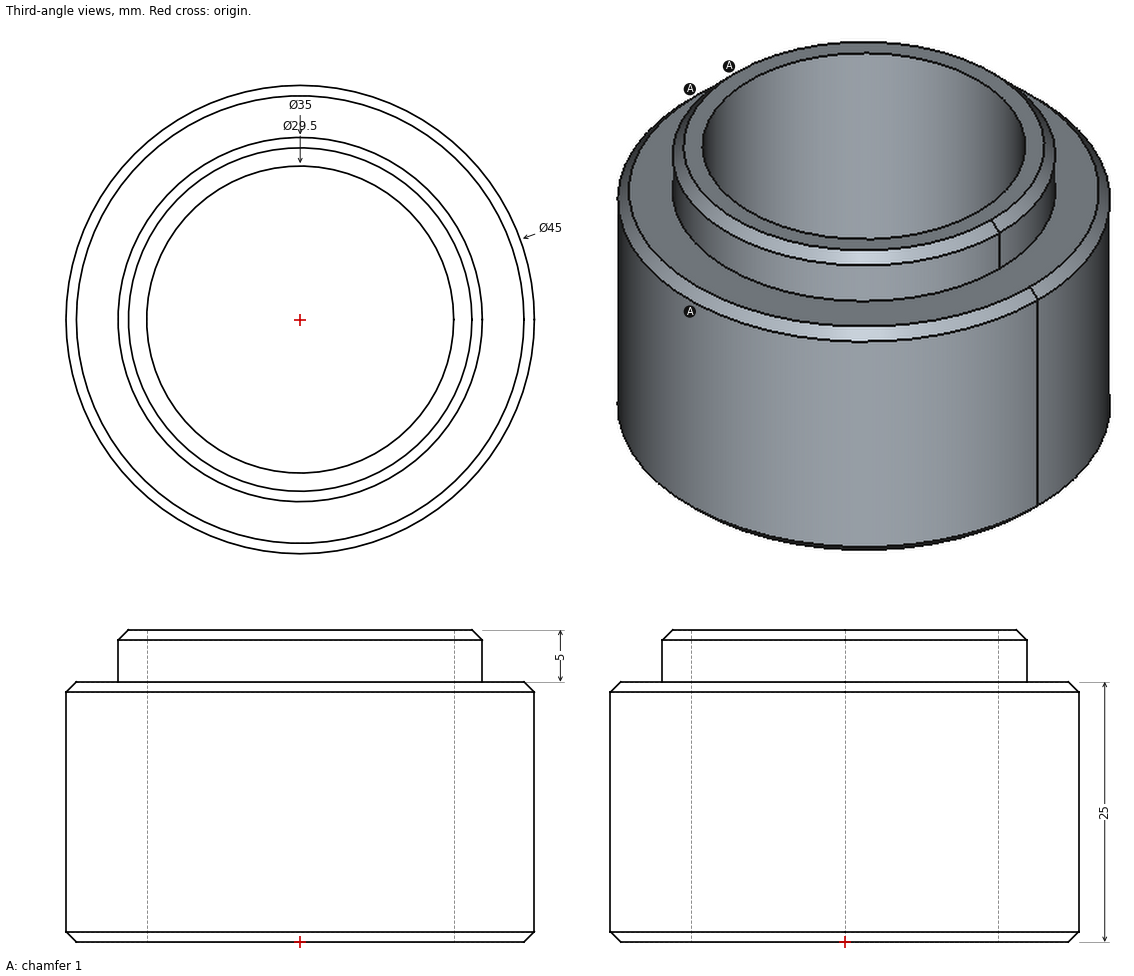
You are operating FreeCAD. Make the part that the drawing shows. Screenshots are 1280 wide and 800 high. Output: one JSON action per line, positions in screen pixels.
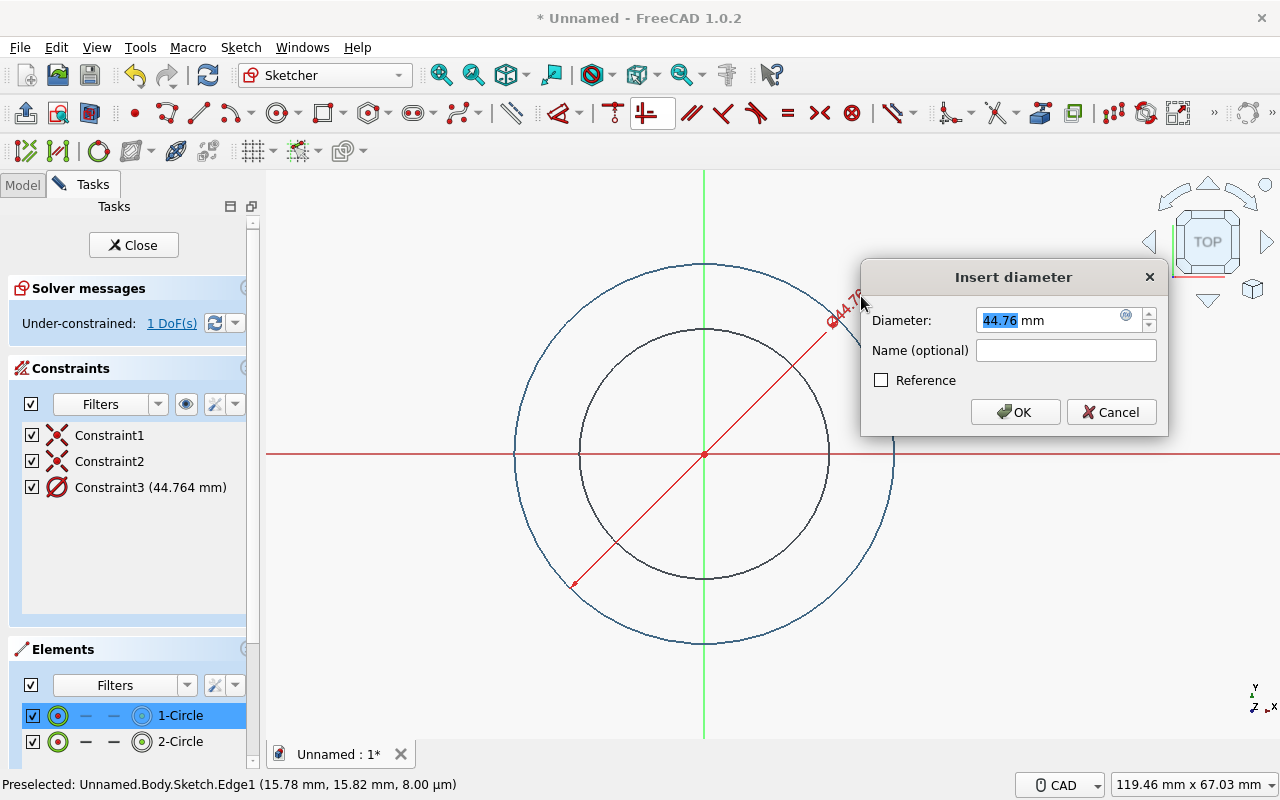
{"action": "type", "text": "45"}
{"action": "key", "text": "Return"}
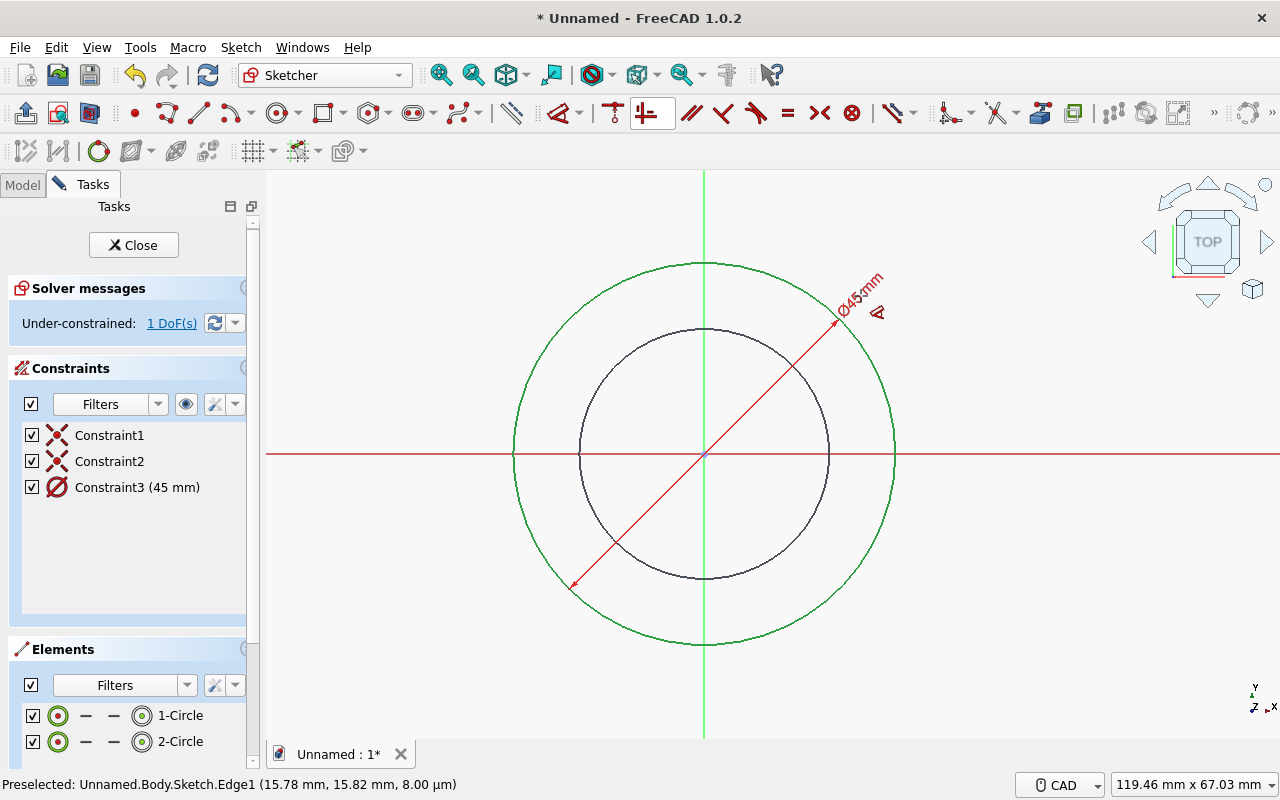
{"action": "left_click", "coordinate": [792, 365]}
{"action": "left_click", "coordinate": [814, 342]}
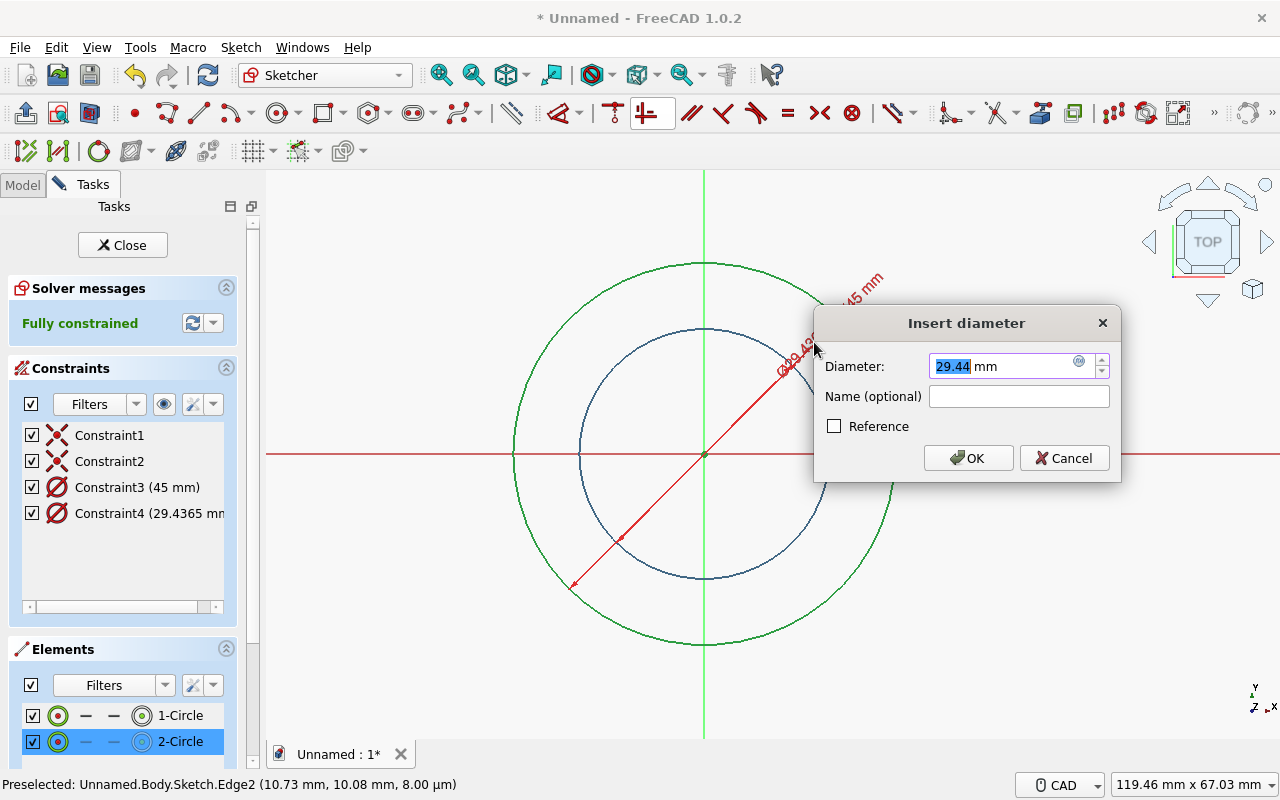
{"action": "type", "text": "29.5"}
{"action": "key", "text": "Return"}
{"action": "key", "text": "Escape"}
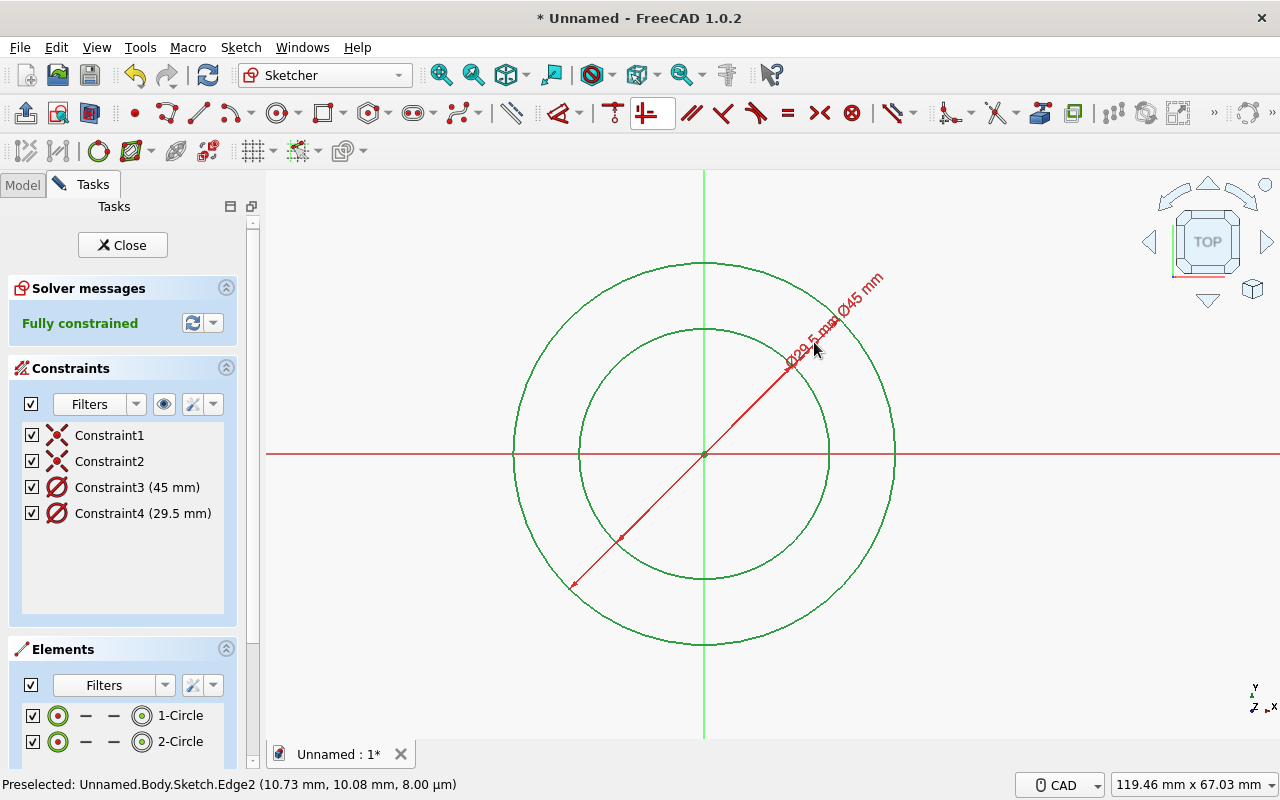
{"action": "left_click", "coordinate": [123, 245]}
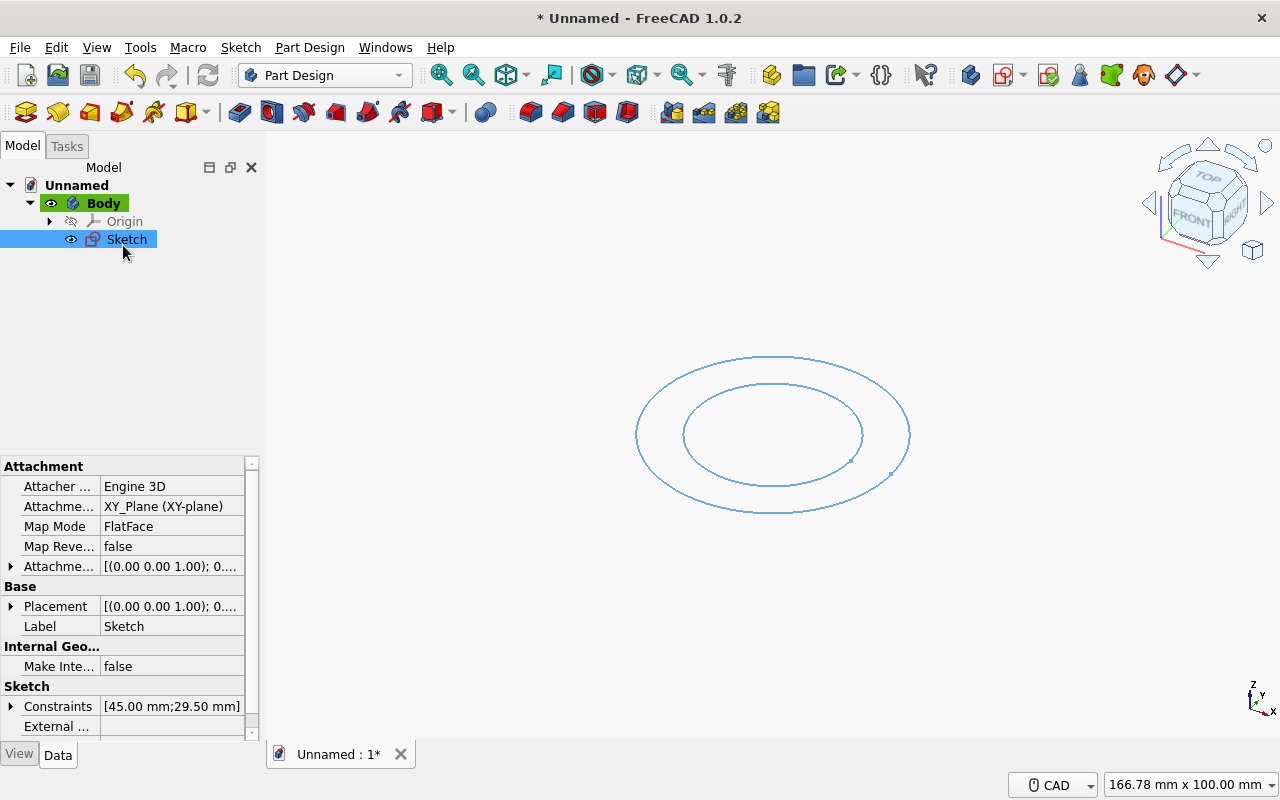
{"action": "left_click", "coordinate": [26, 112]}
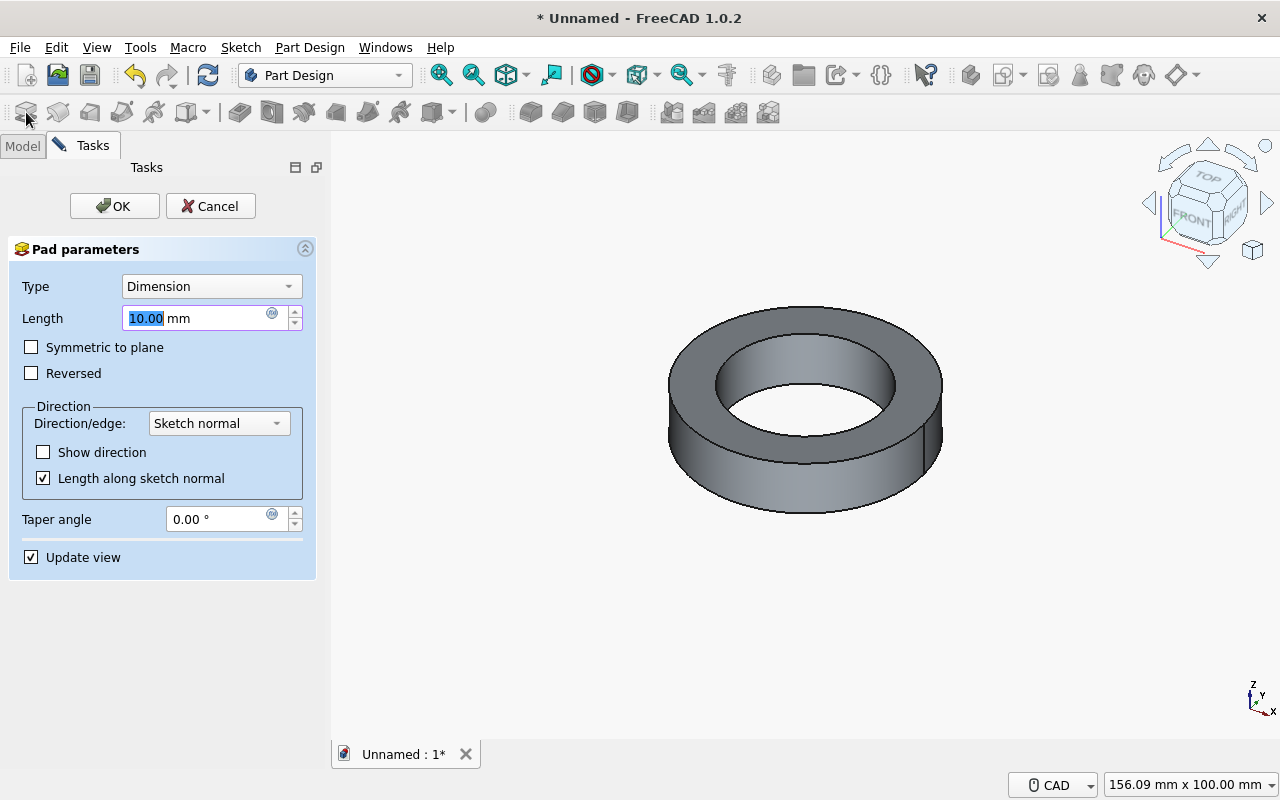
{"action": "type", "text": "25"}
{"action": "key", "text": "Tab"}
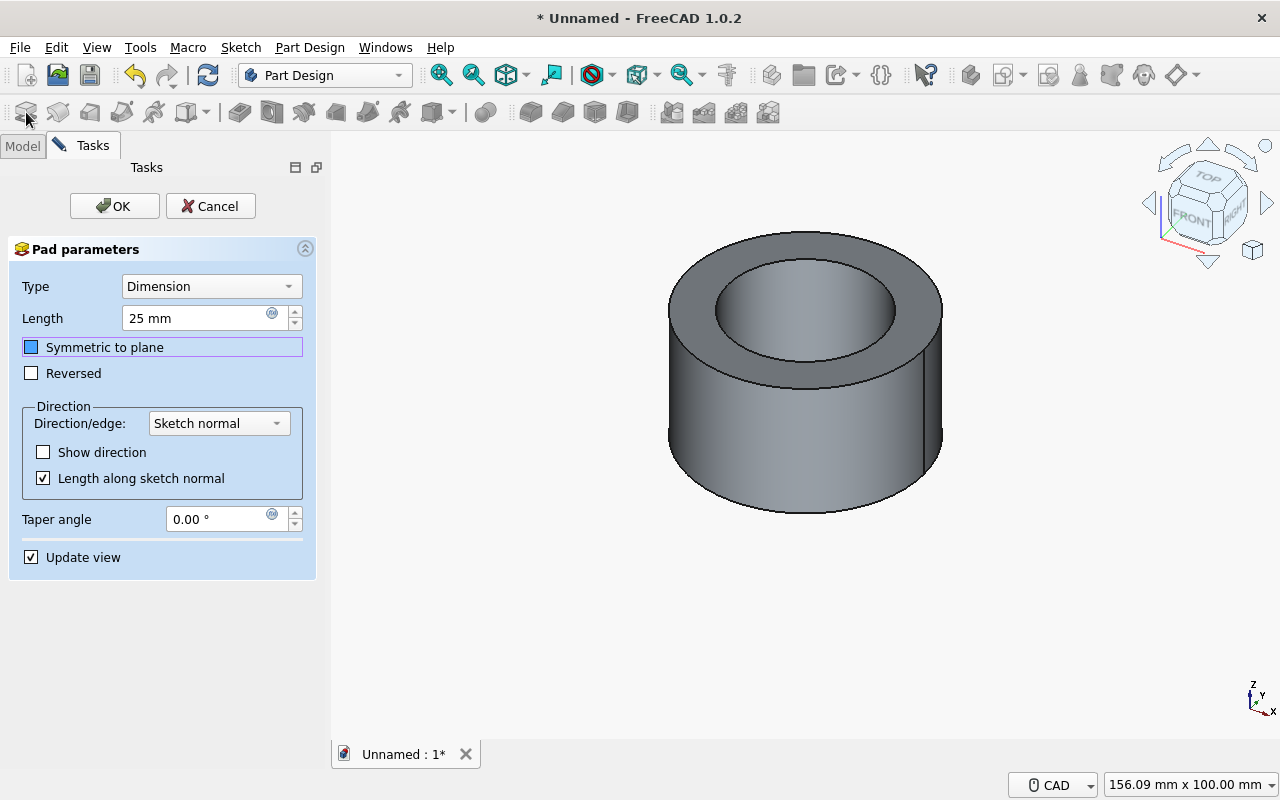
{"action": "left_click", "coordinate": [115, 206]}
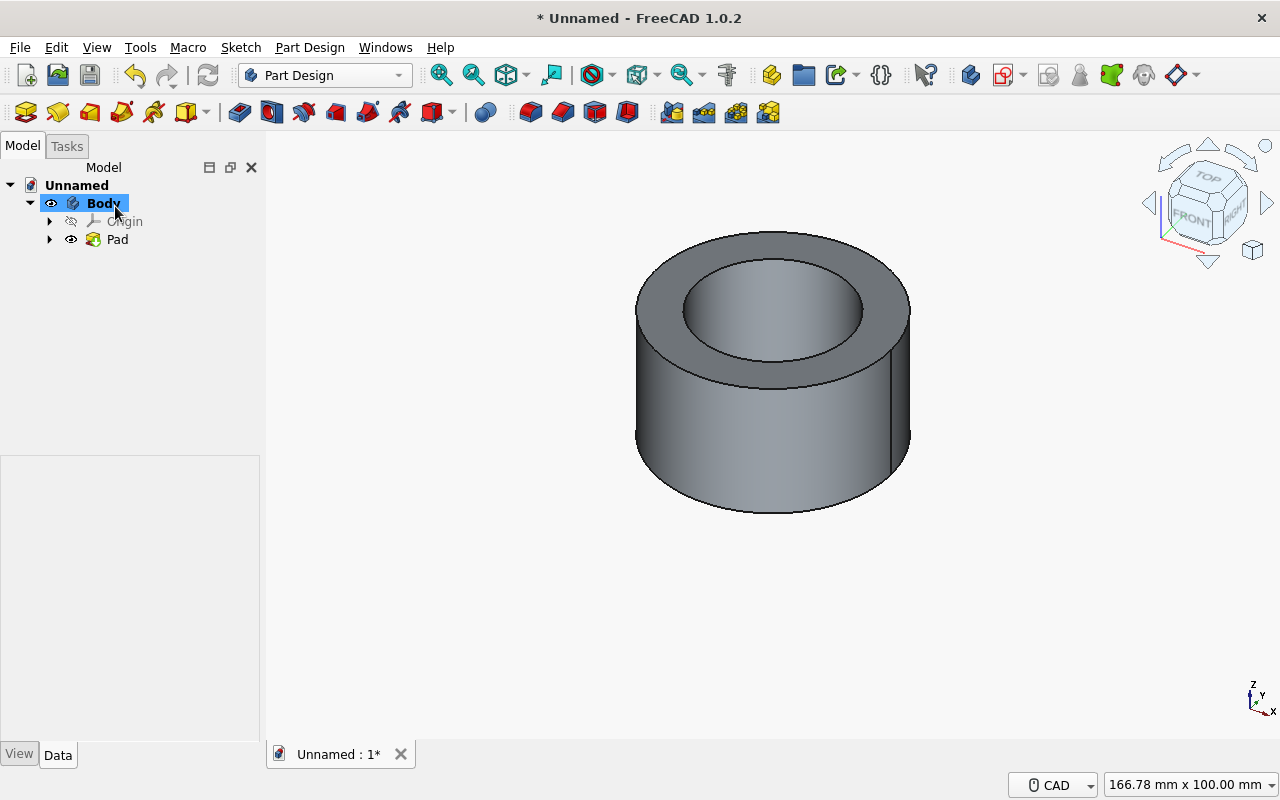
{"action": "left_click", "coordinate": [666, 326]}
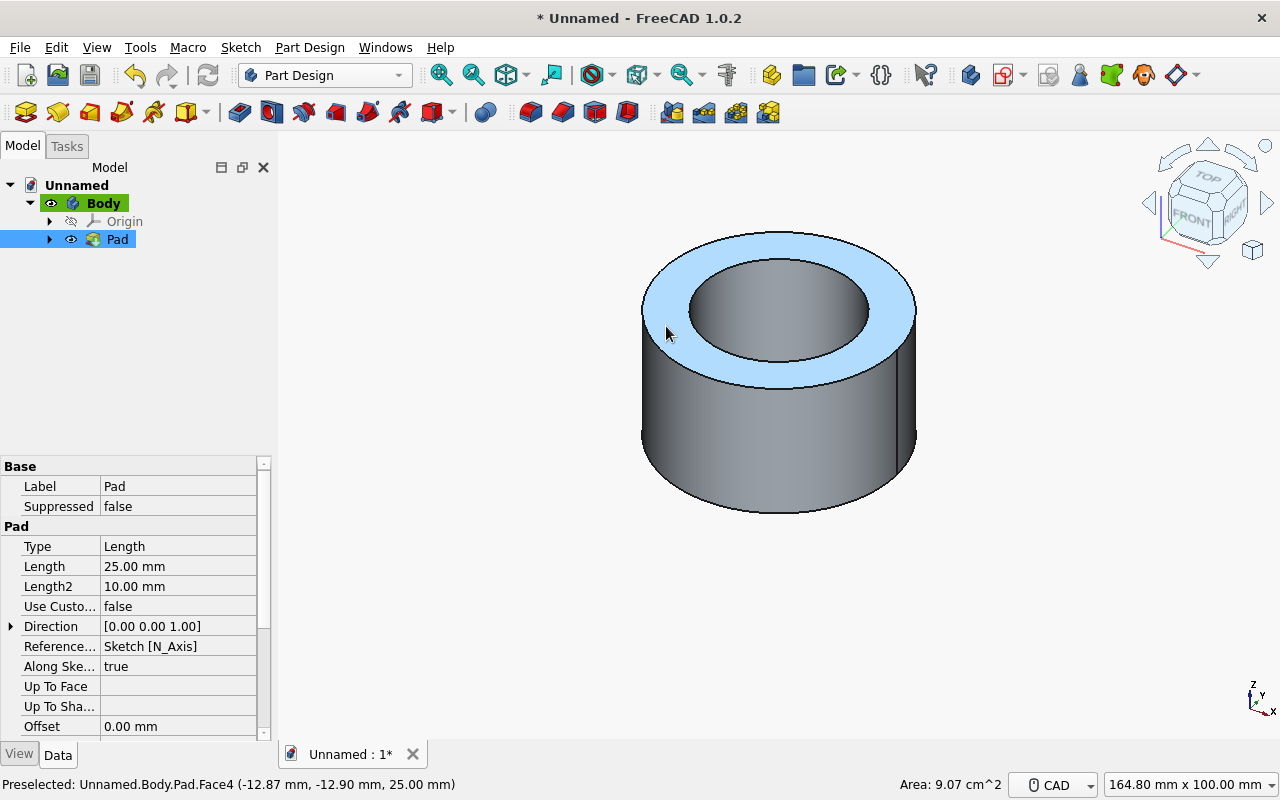
{"action": "left_click", "coordinate": [1004, 76]}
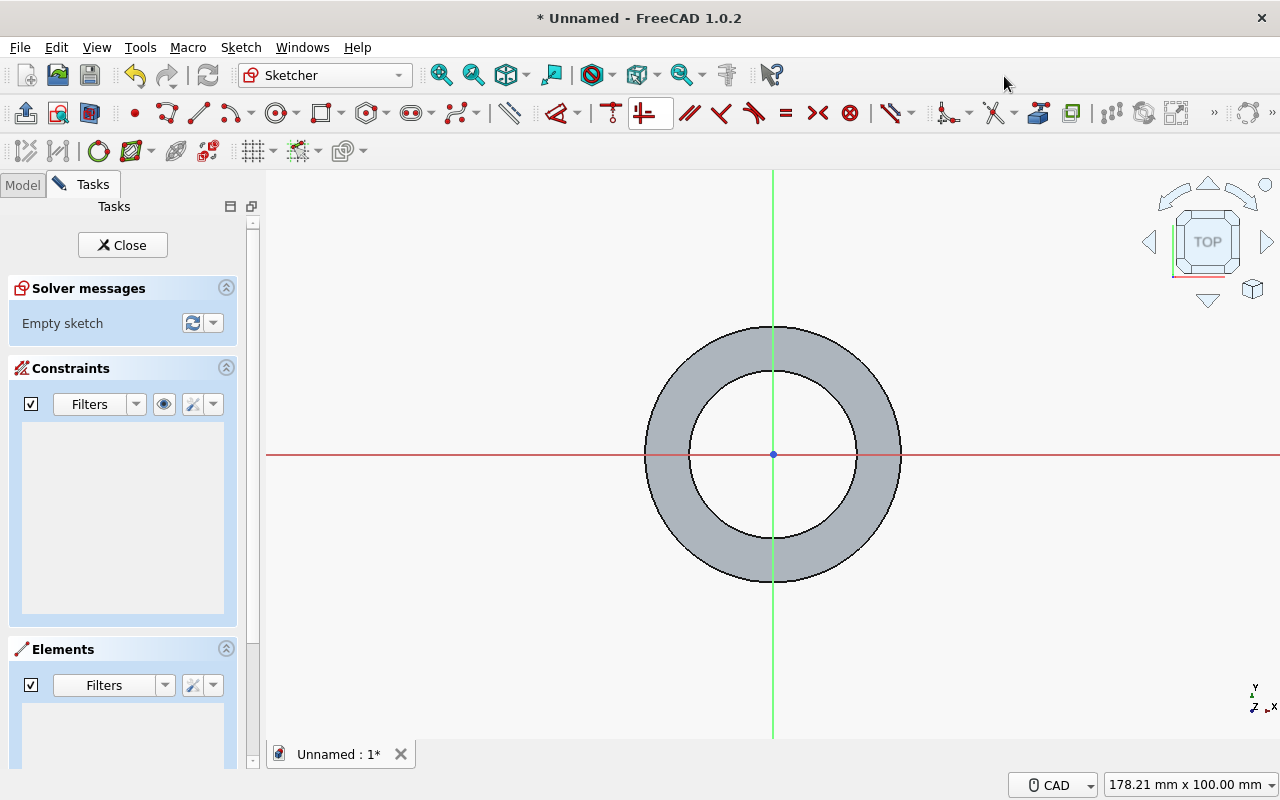
{"action": "scroll", "coordinate": [856, 454], "scroll_direction": "up", "scroll_amount": 3}